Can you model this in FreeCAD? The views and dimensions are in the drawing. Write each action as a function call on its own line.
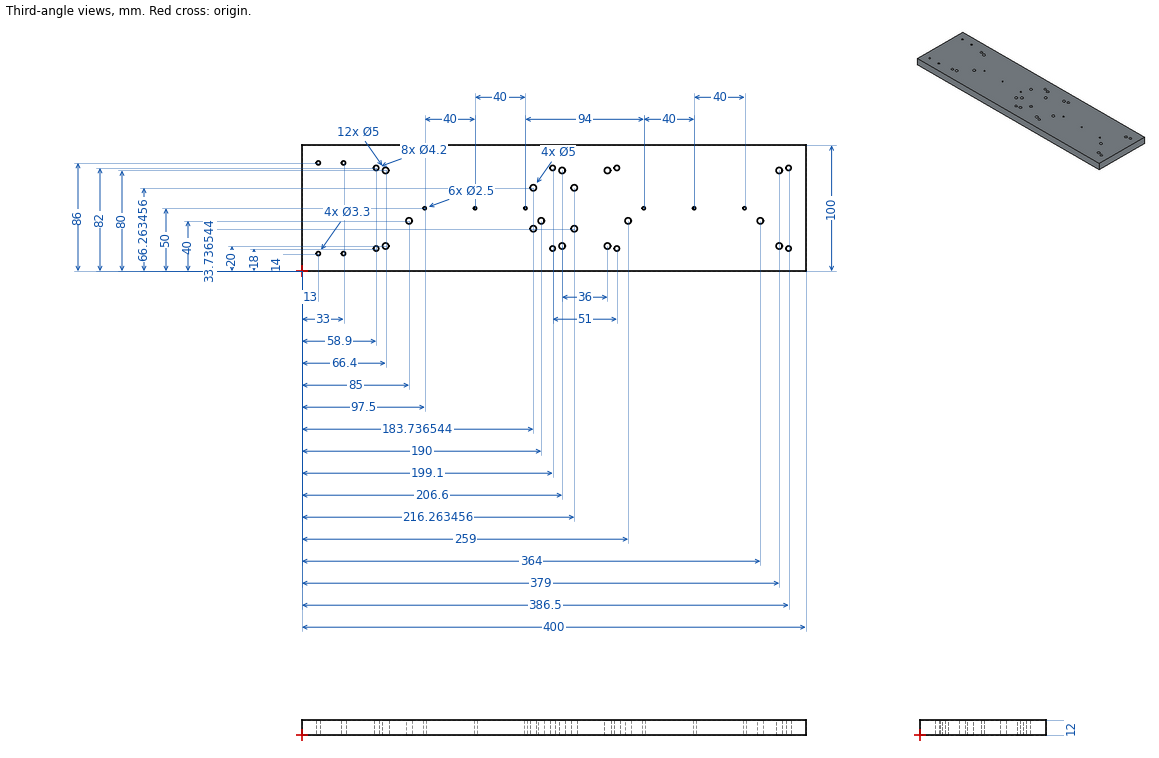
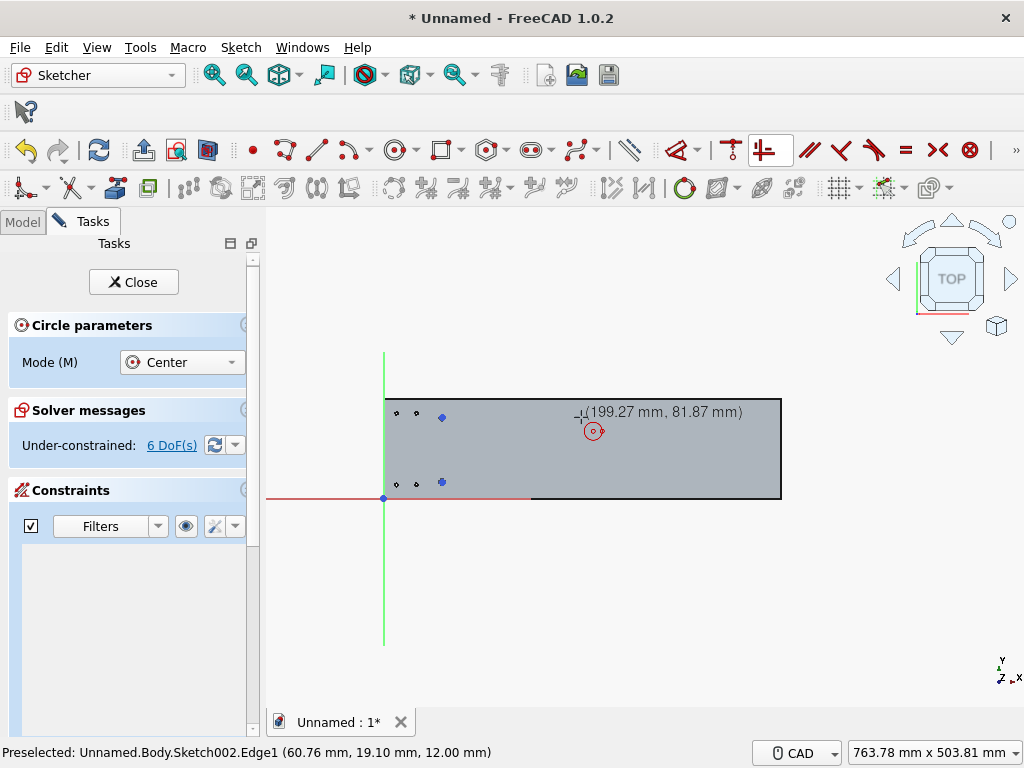
click(581, 417)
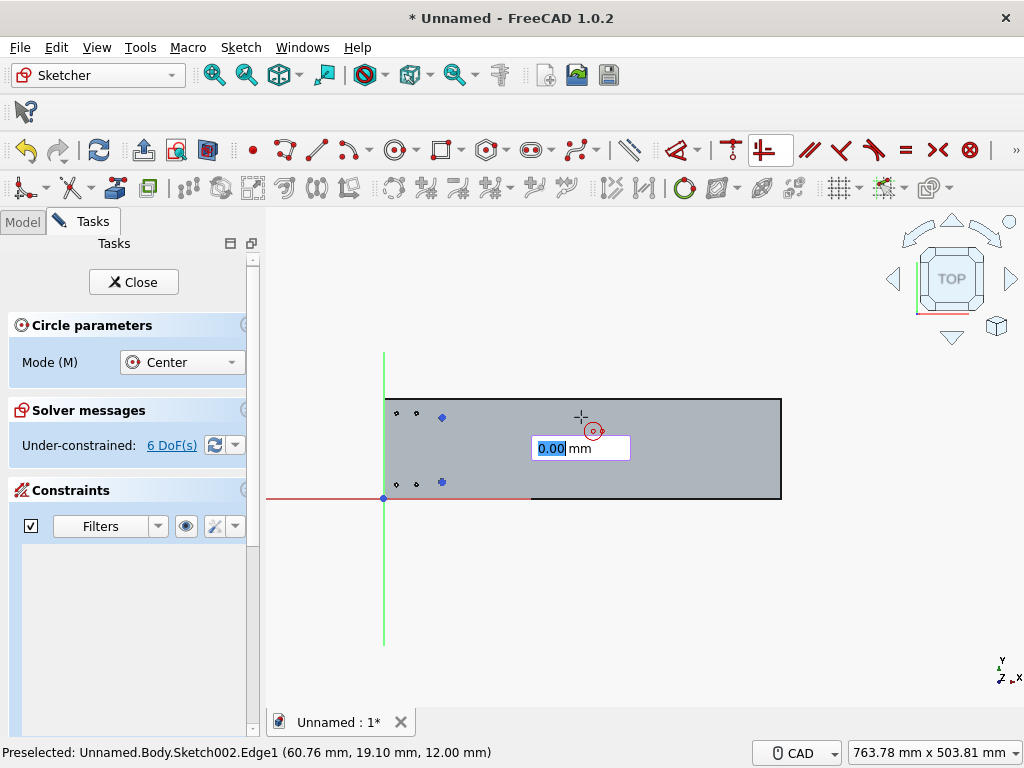
scroll(583, 416, up, 11)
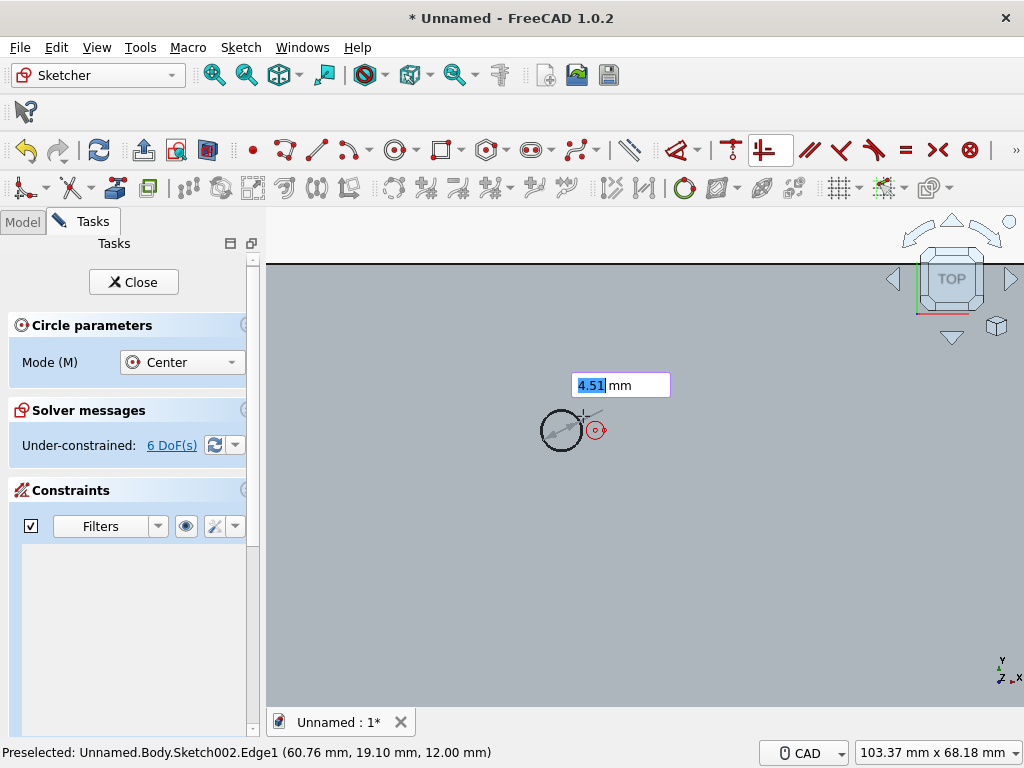
click(577, 411)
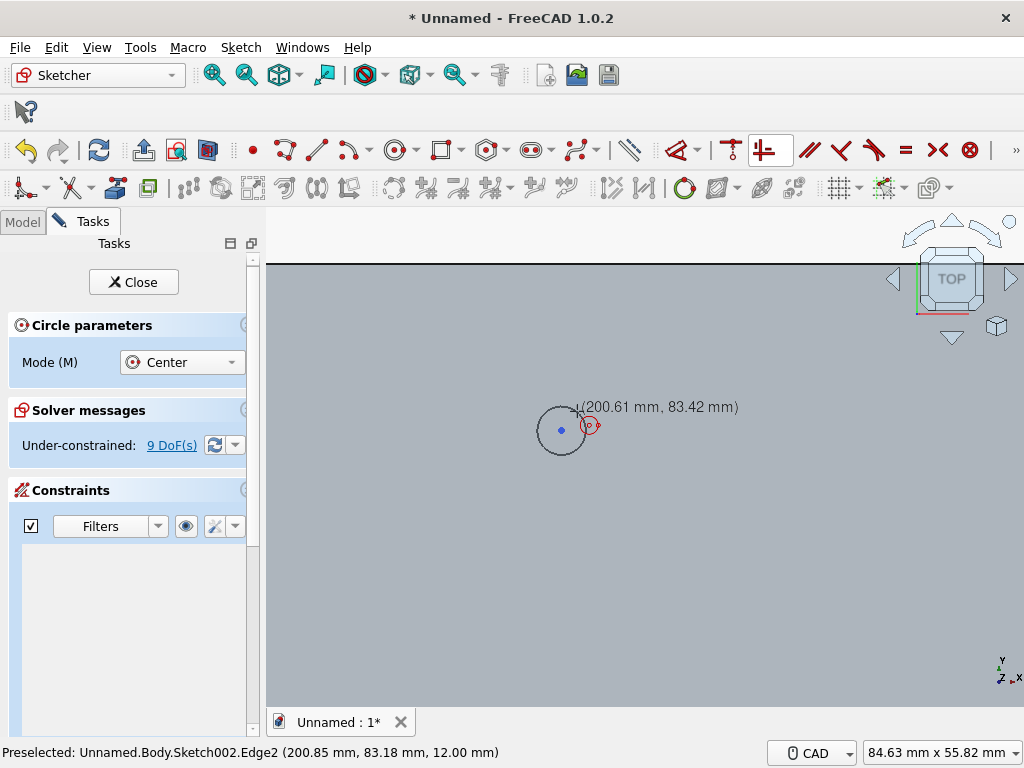
scroll(583, 416, down, 11)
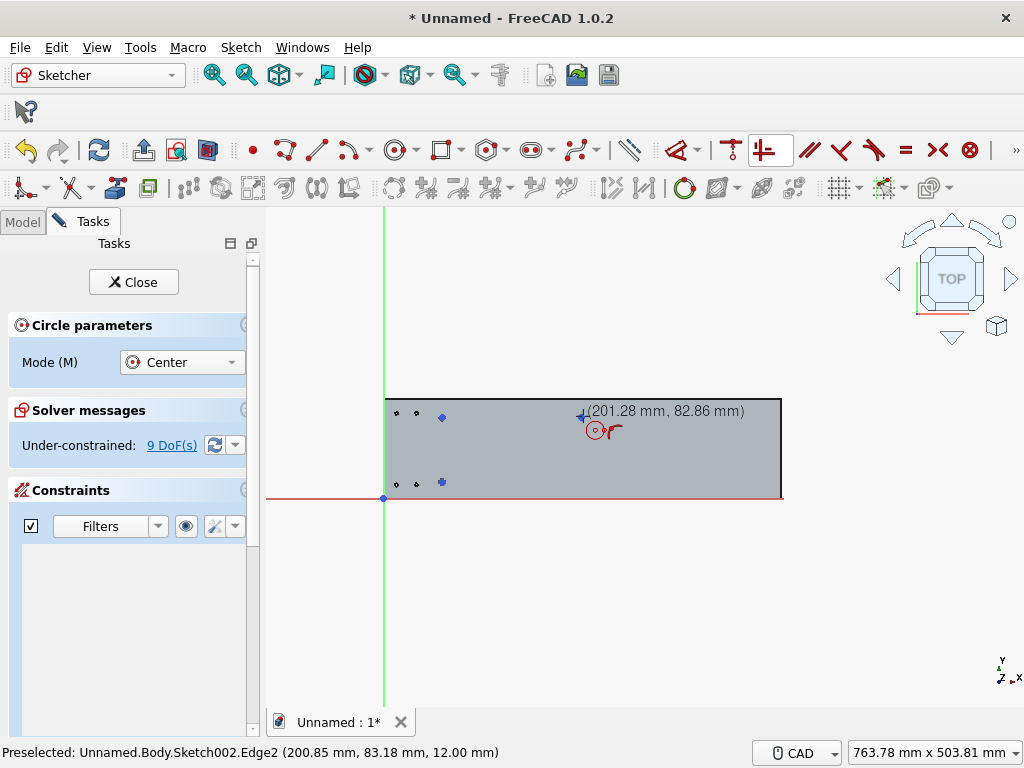
scroll(581, 481, up, 12)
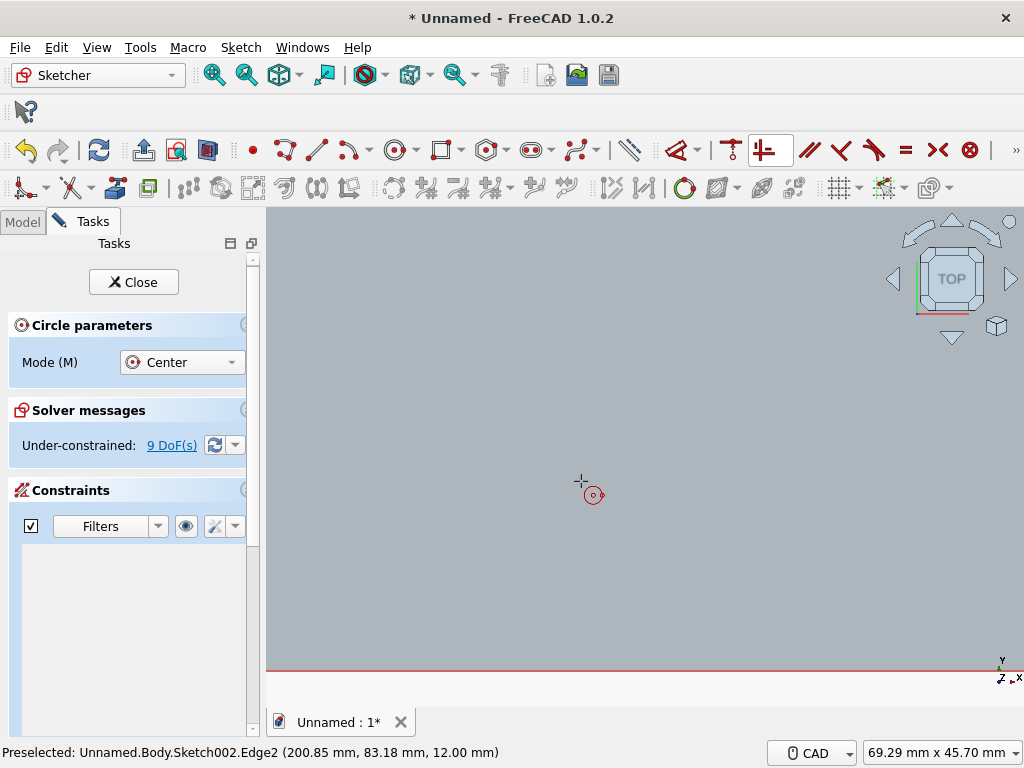
scroll(581, 482, down, 12)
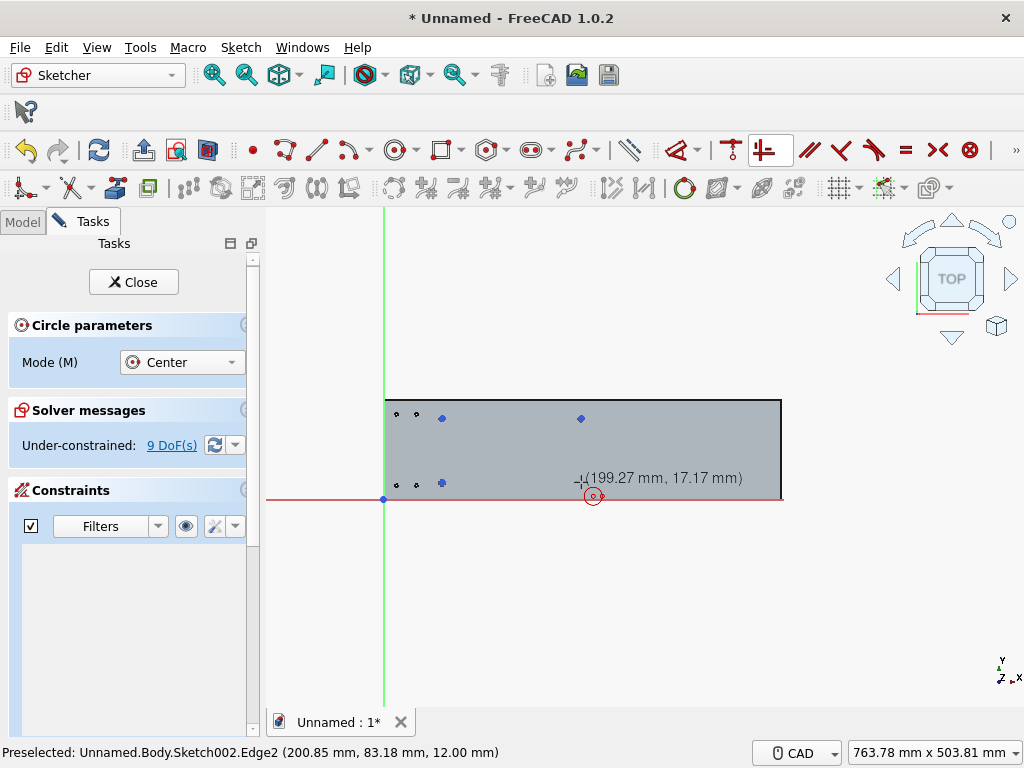
click(581, 482)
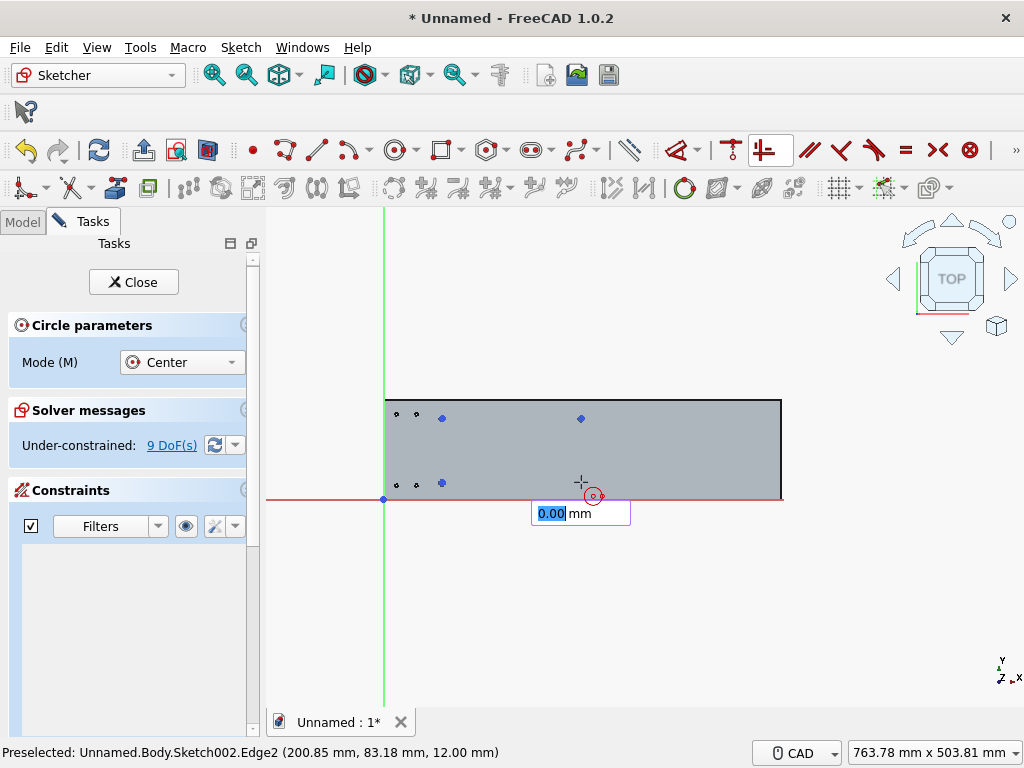
scroll(583, 480, up, 11)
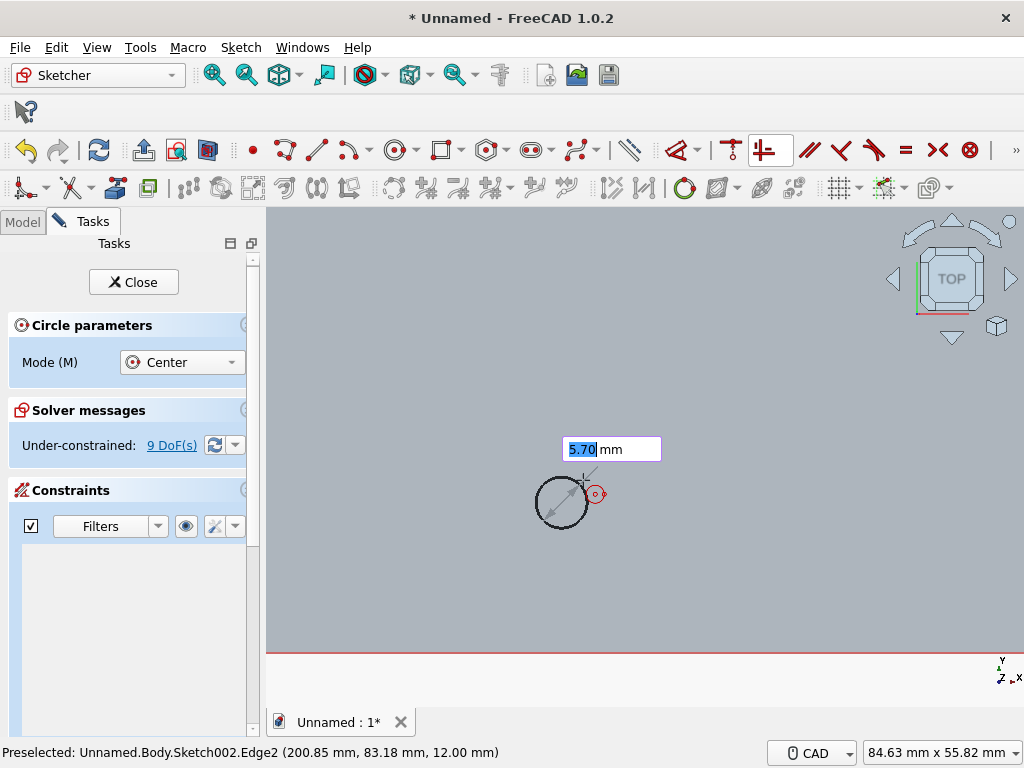
click(577, 478)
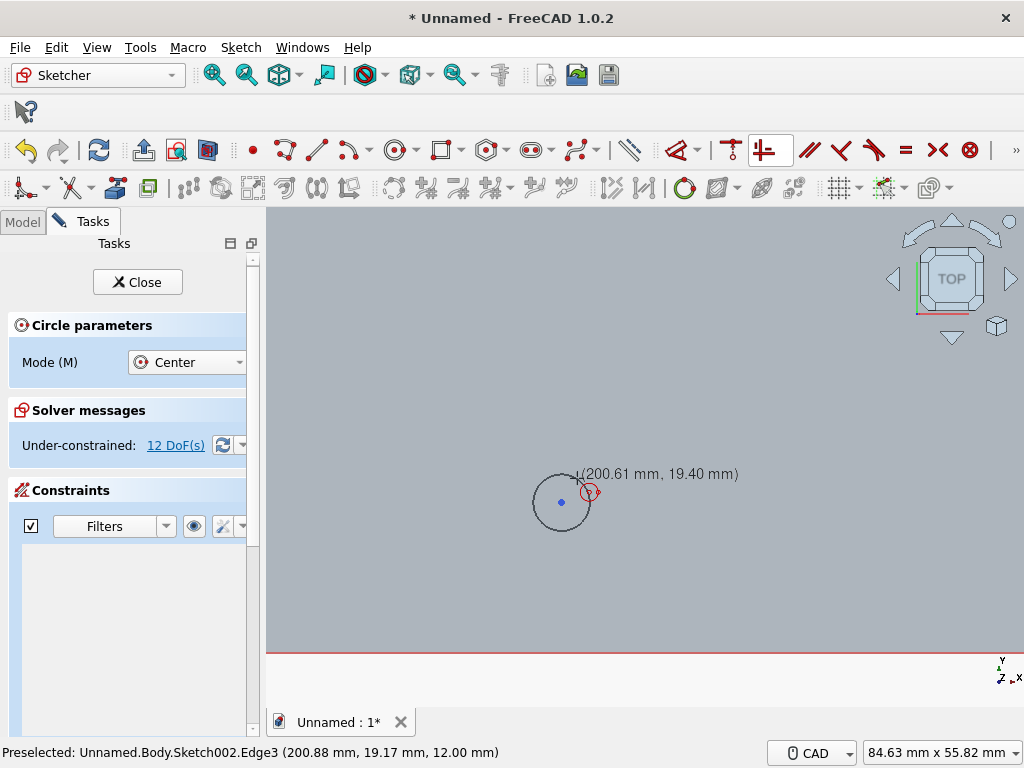
scroll(583, 480, down, 11)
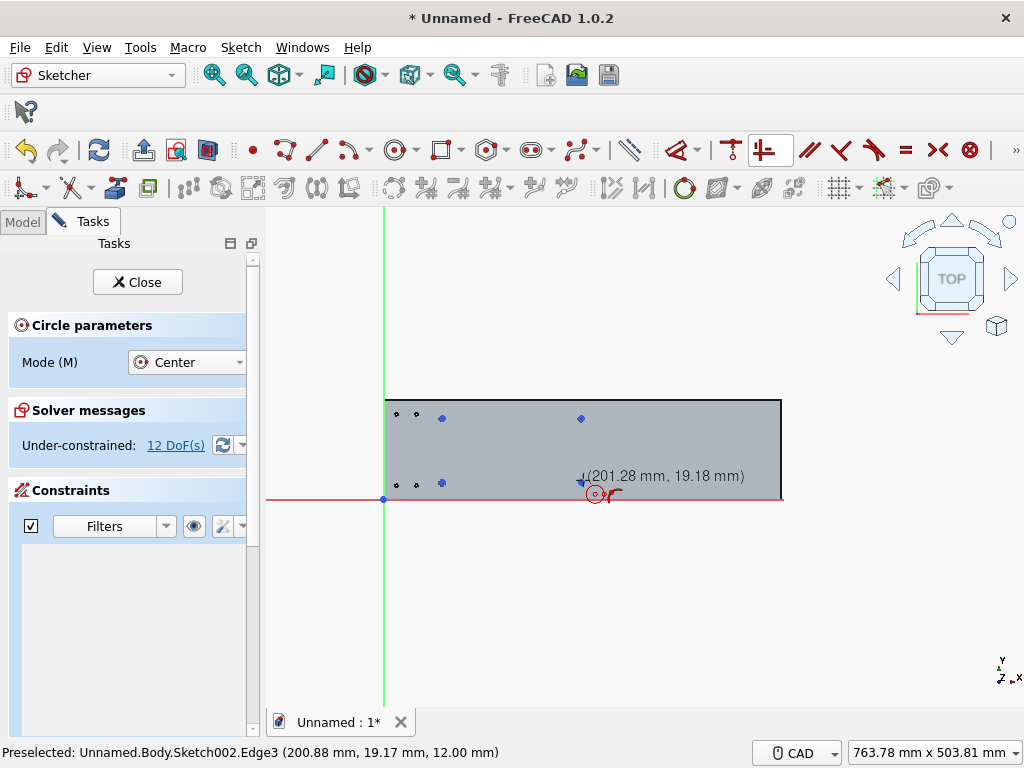
scroll(632, 482, up, 12)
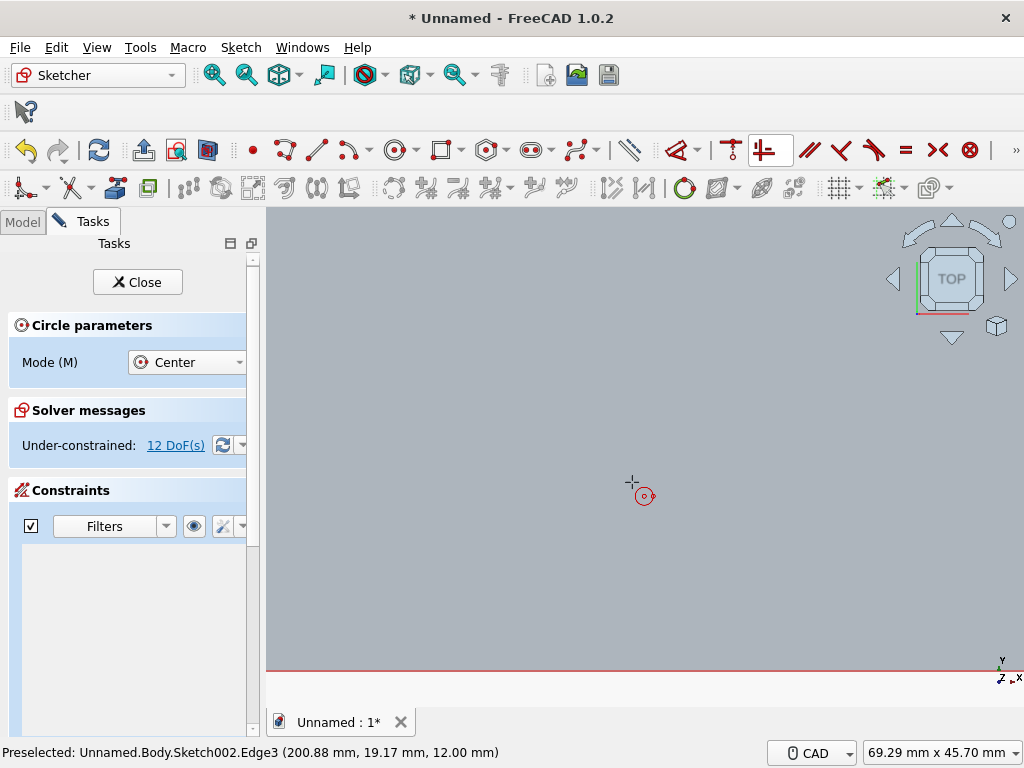
scroll(633, 482, down, 12)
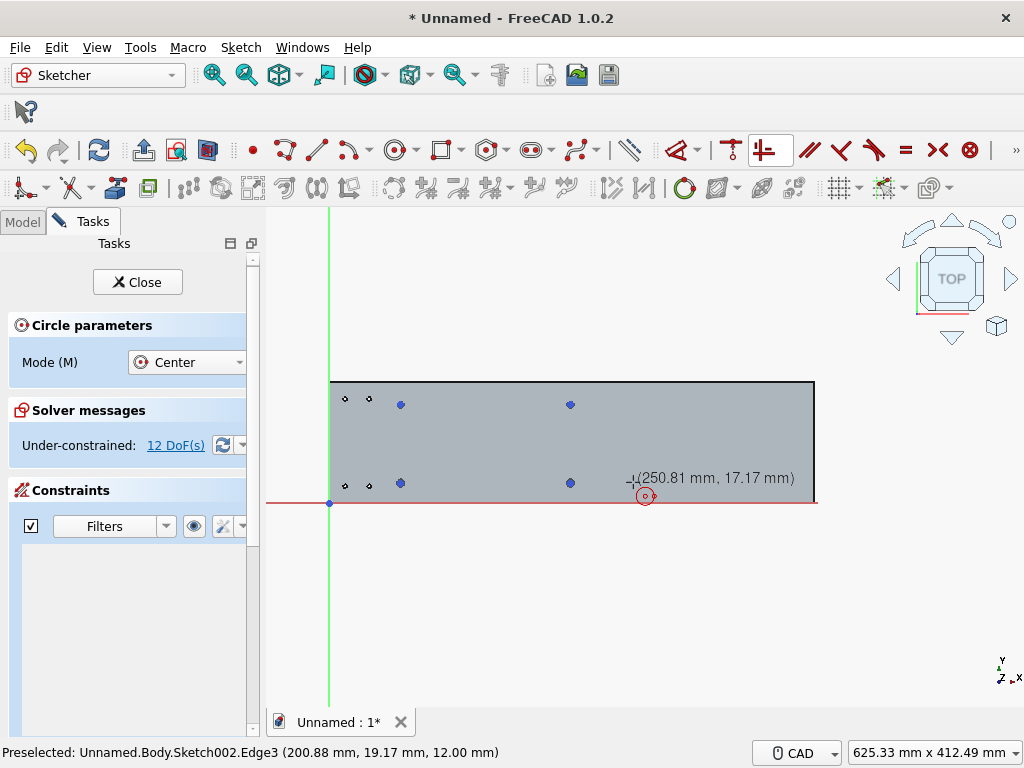
click(633, 482)